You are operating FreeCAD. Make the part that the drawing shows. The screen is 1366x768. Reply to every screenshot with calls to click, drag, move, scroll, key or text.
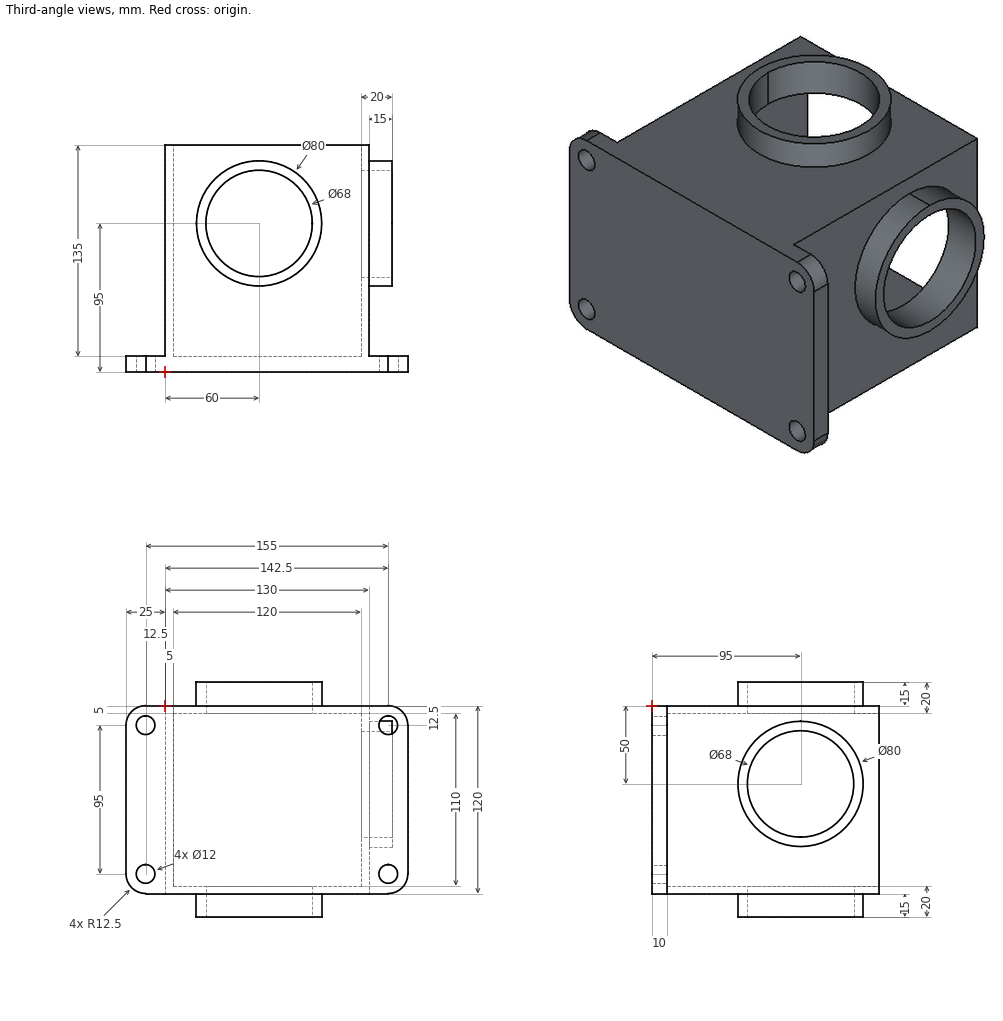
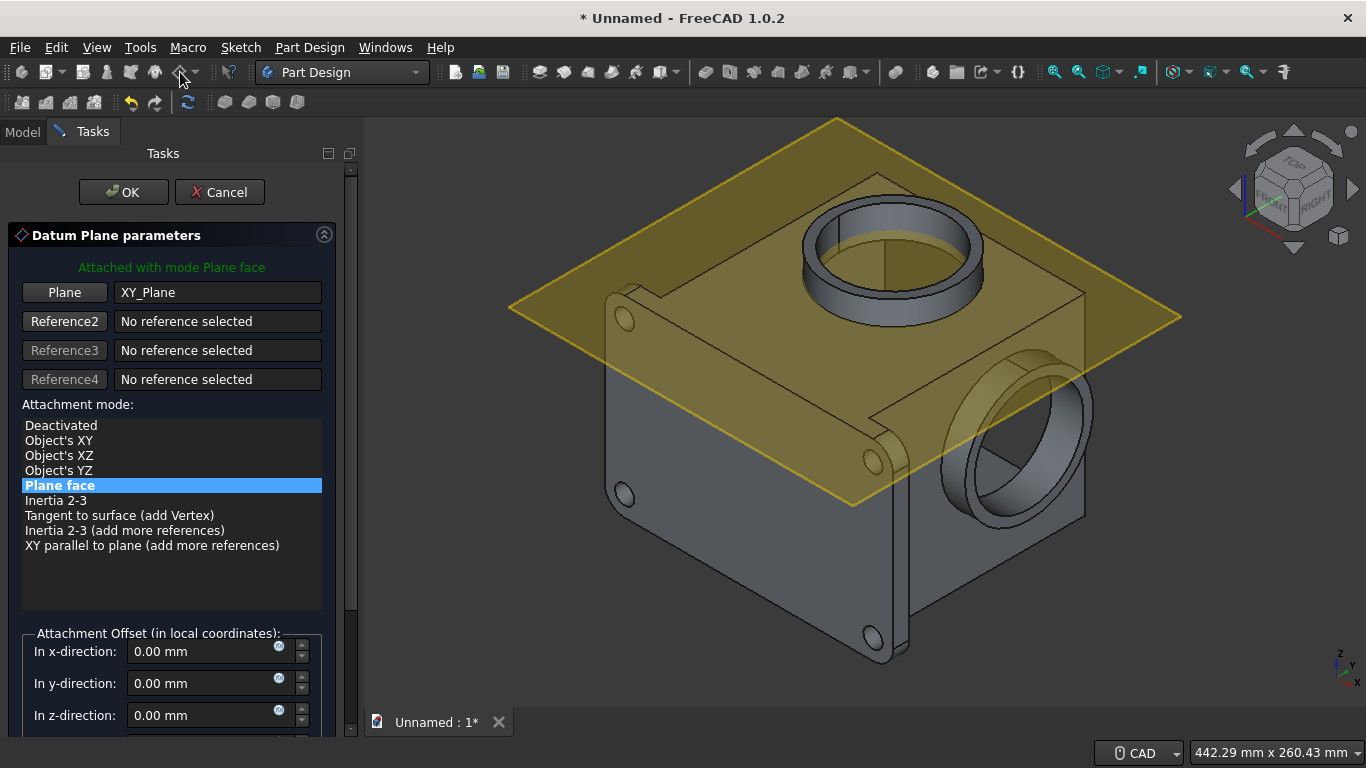
triple_click(210, 715)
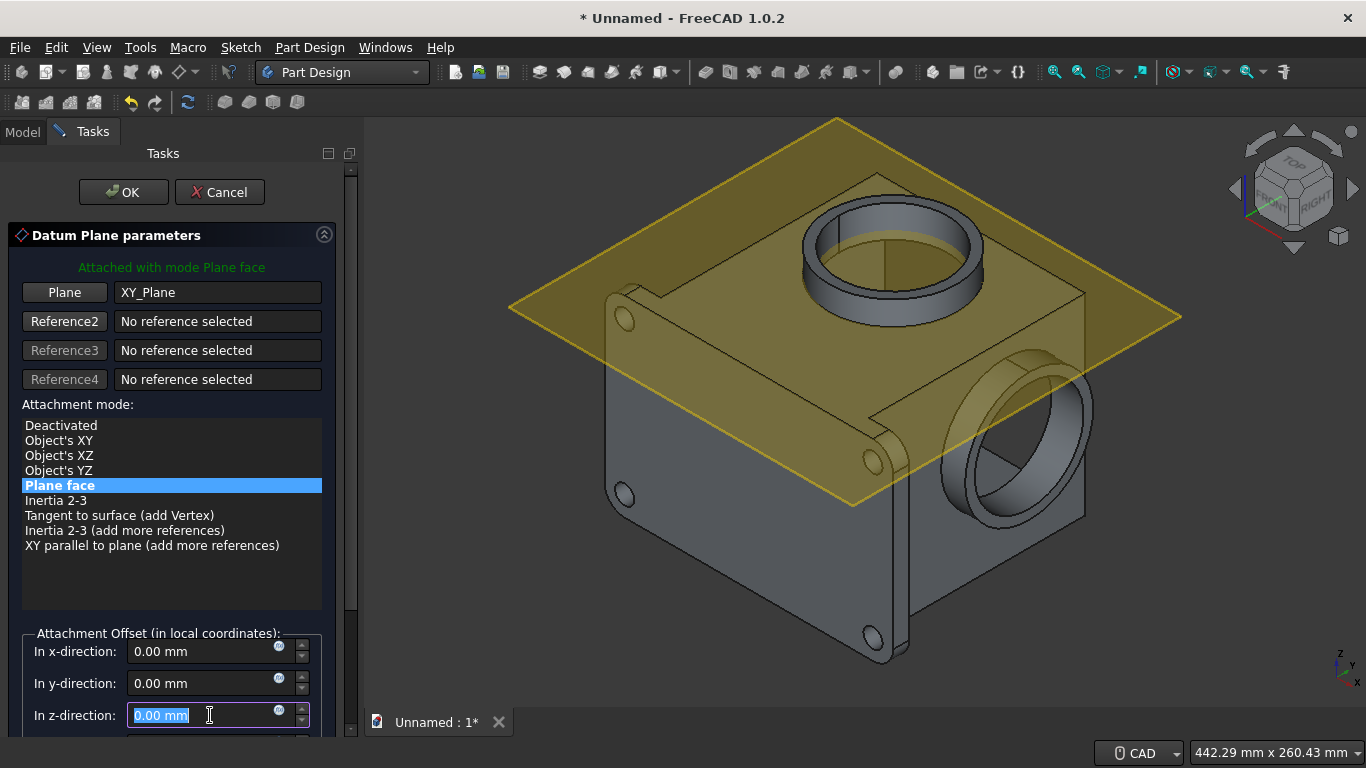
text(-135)
key(Tab)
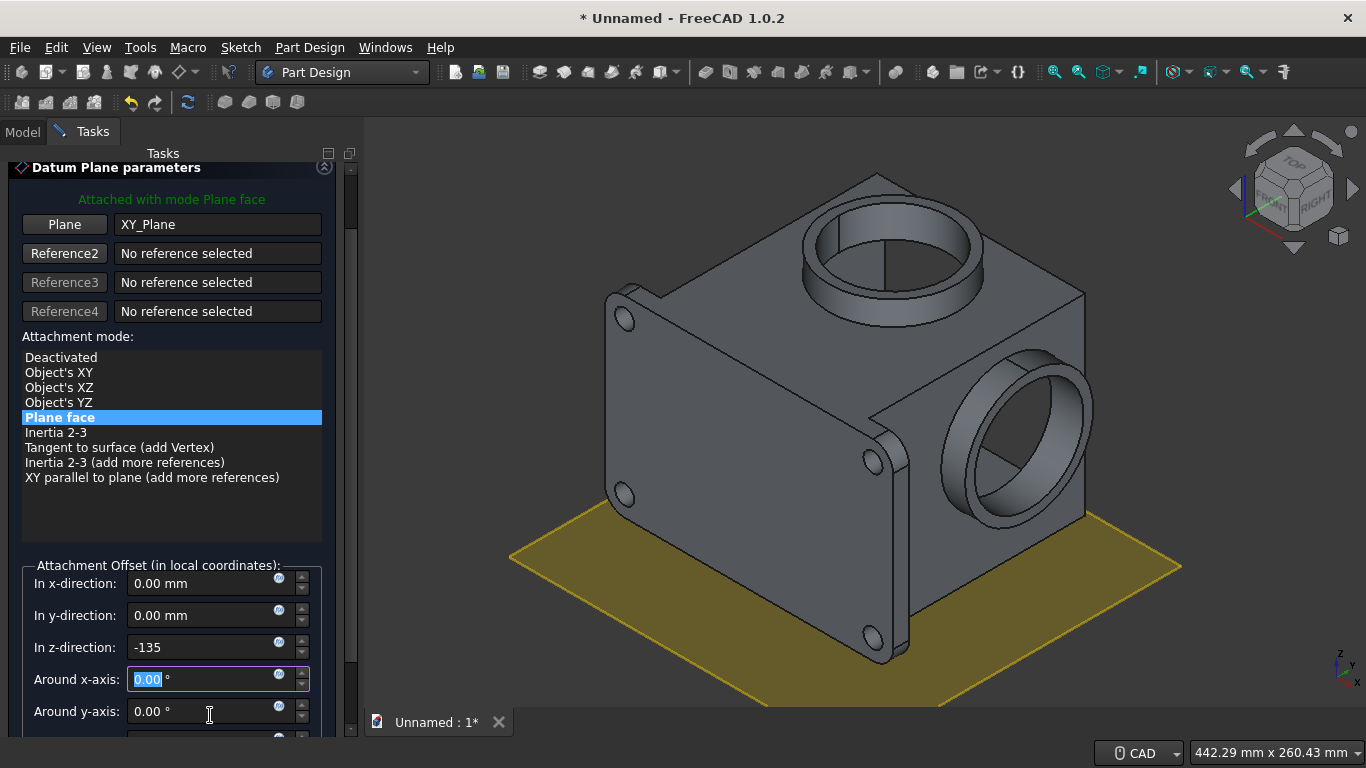
scroll(351, 450, up, 2)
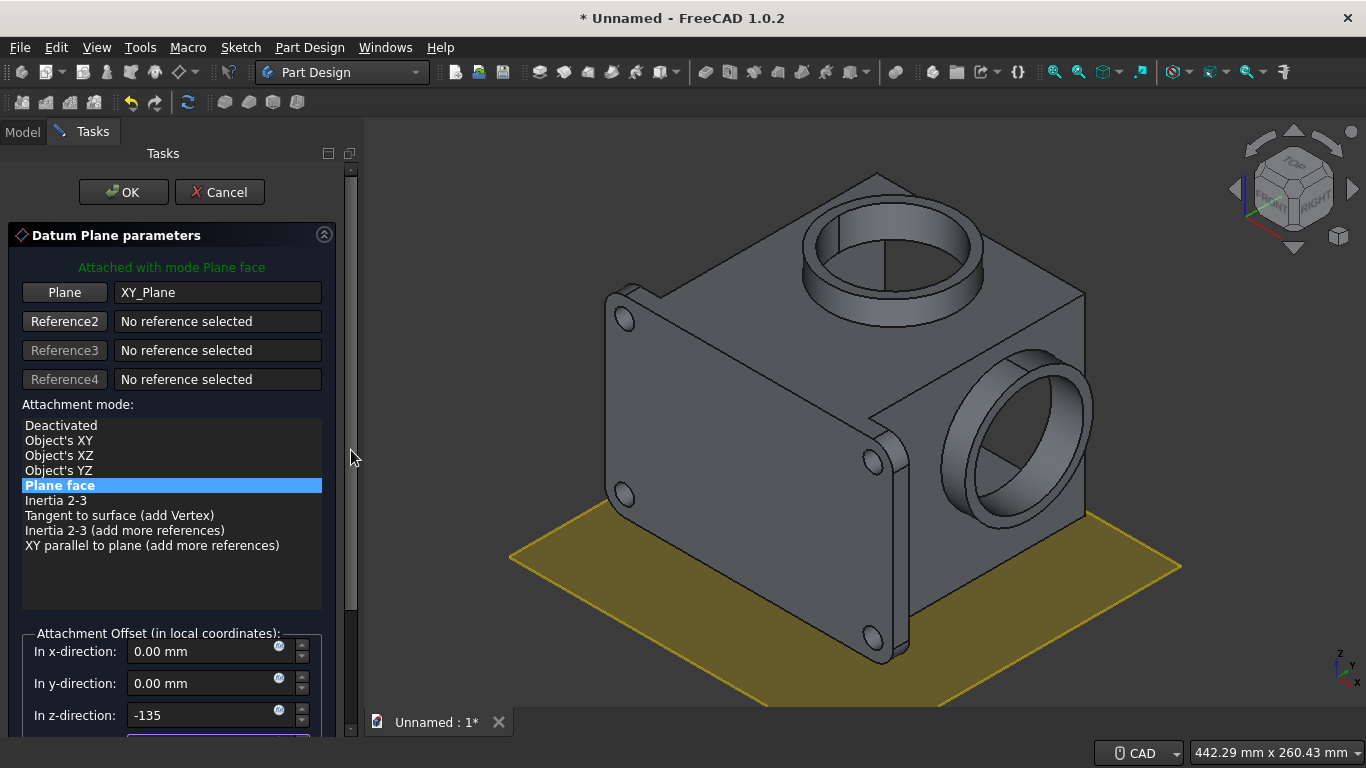
click(124, 192)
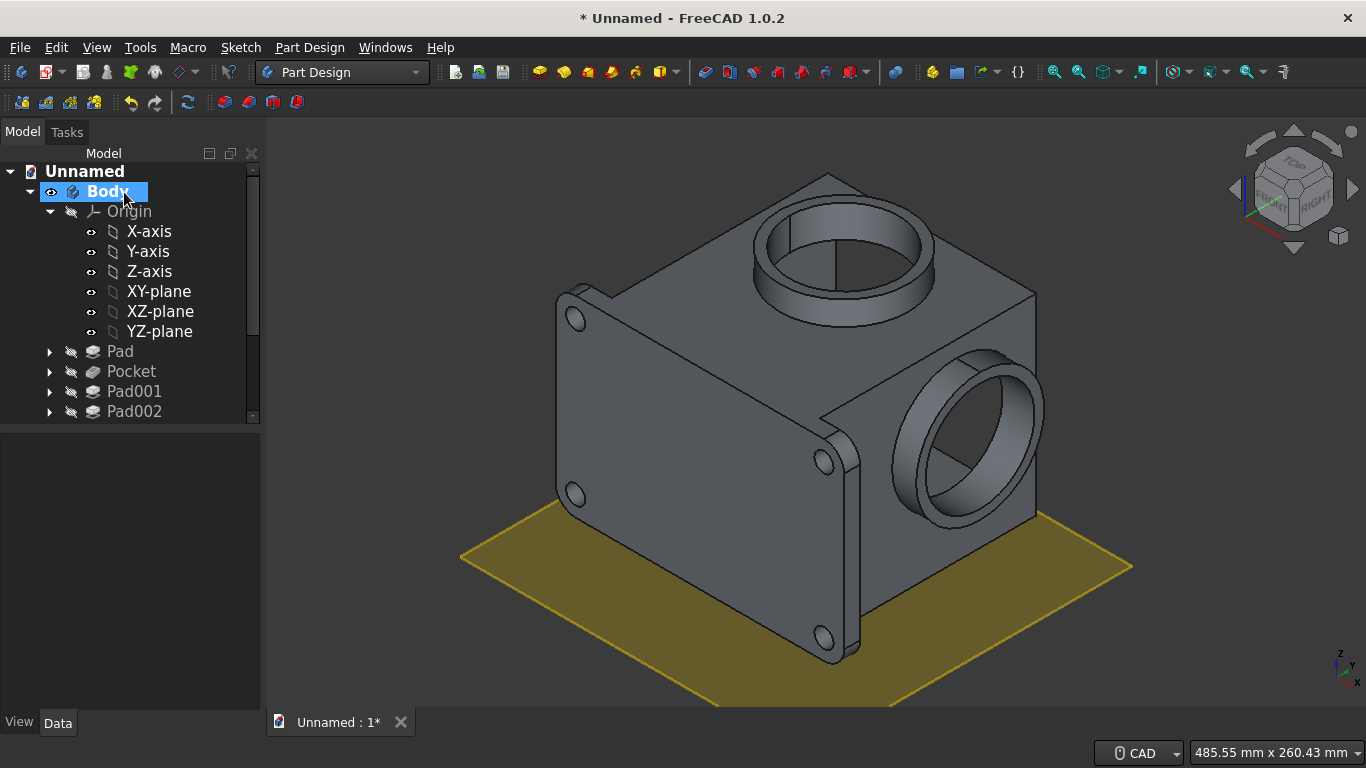
scroll(100, 287, down, 3)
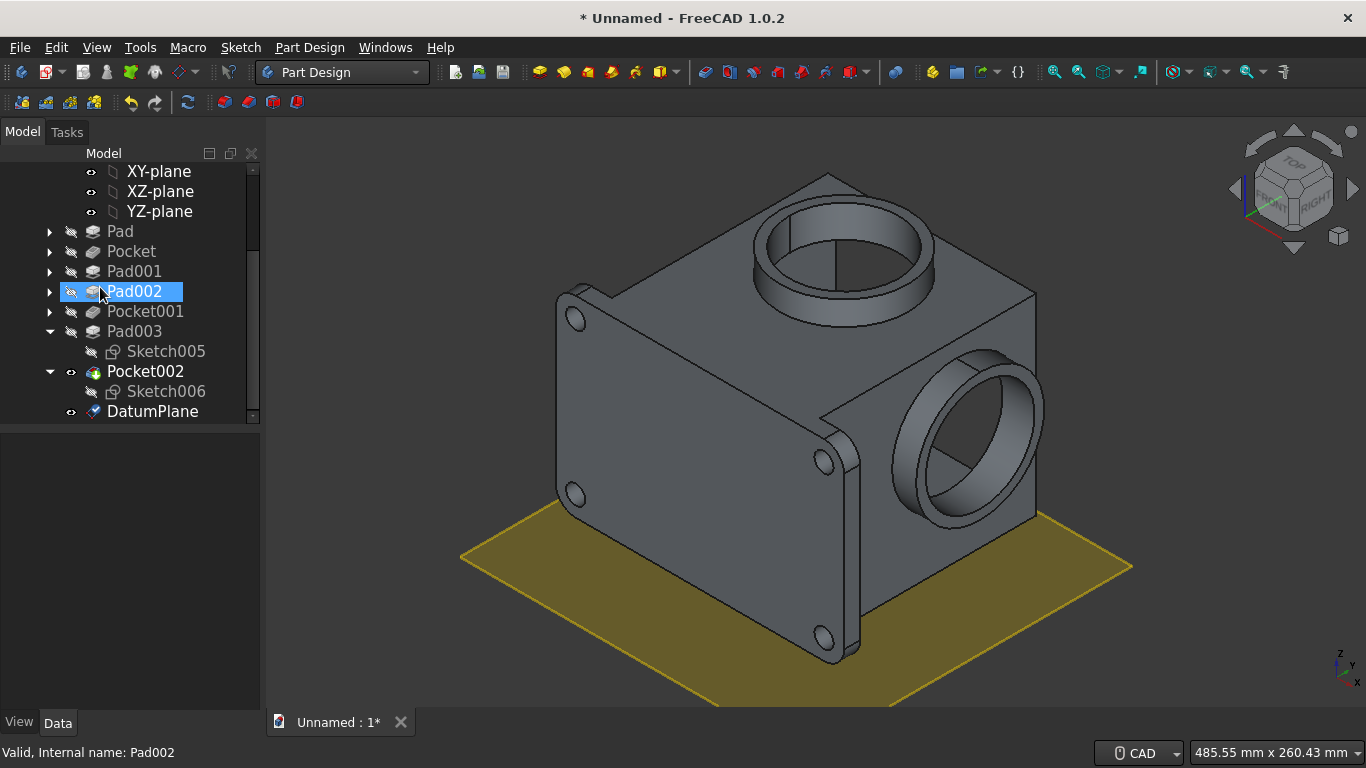
click(116, 412)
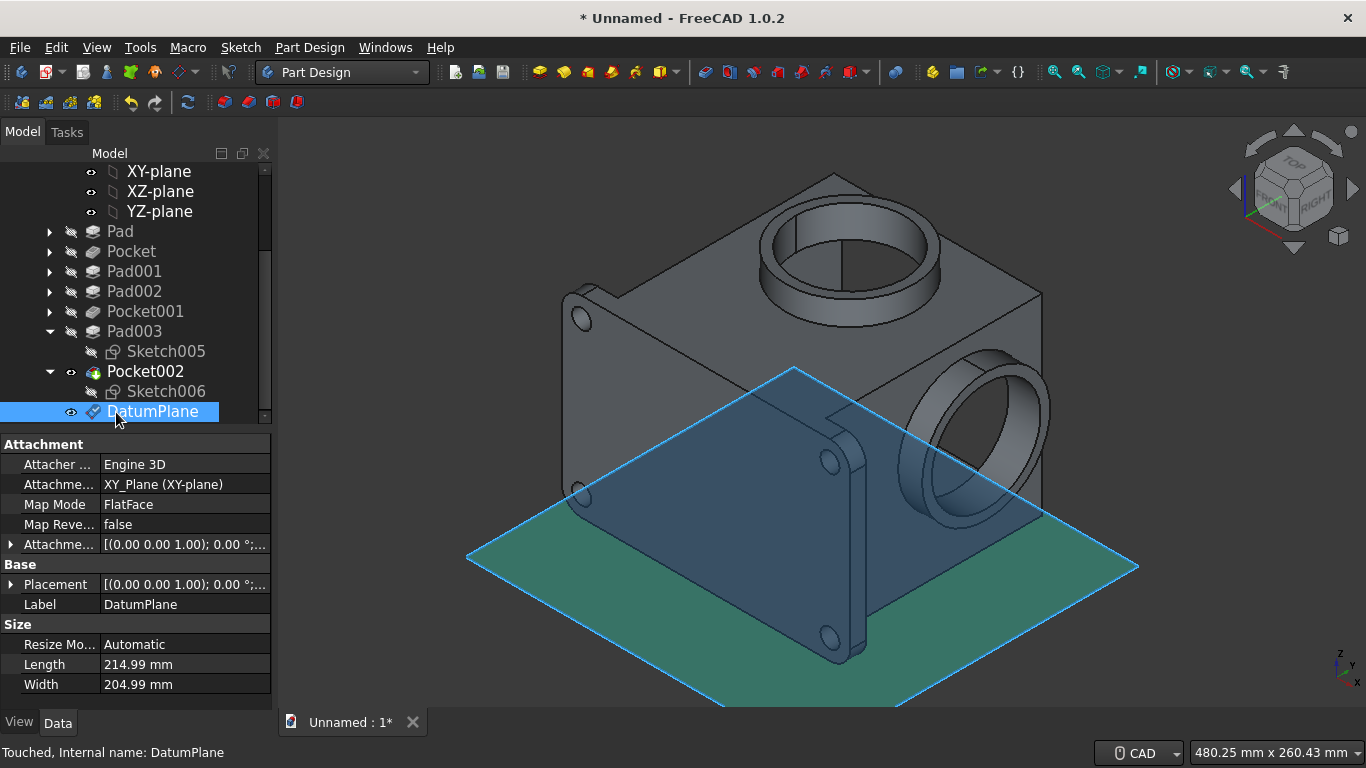
click(46, 72)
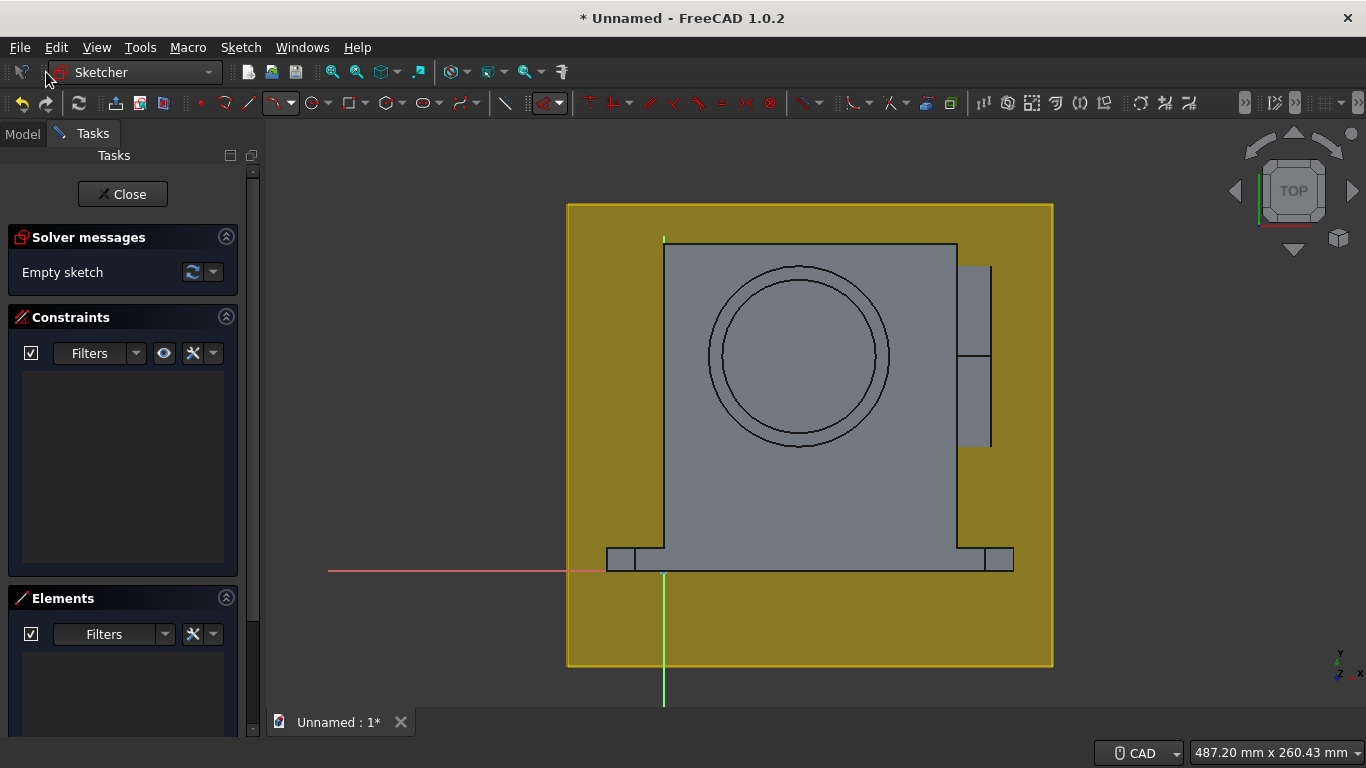
click(164, 104)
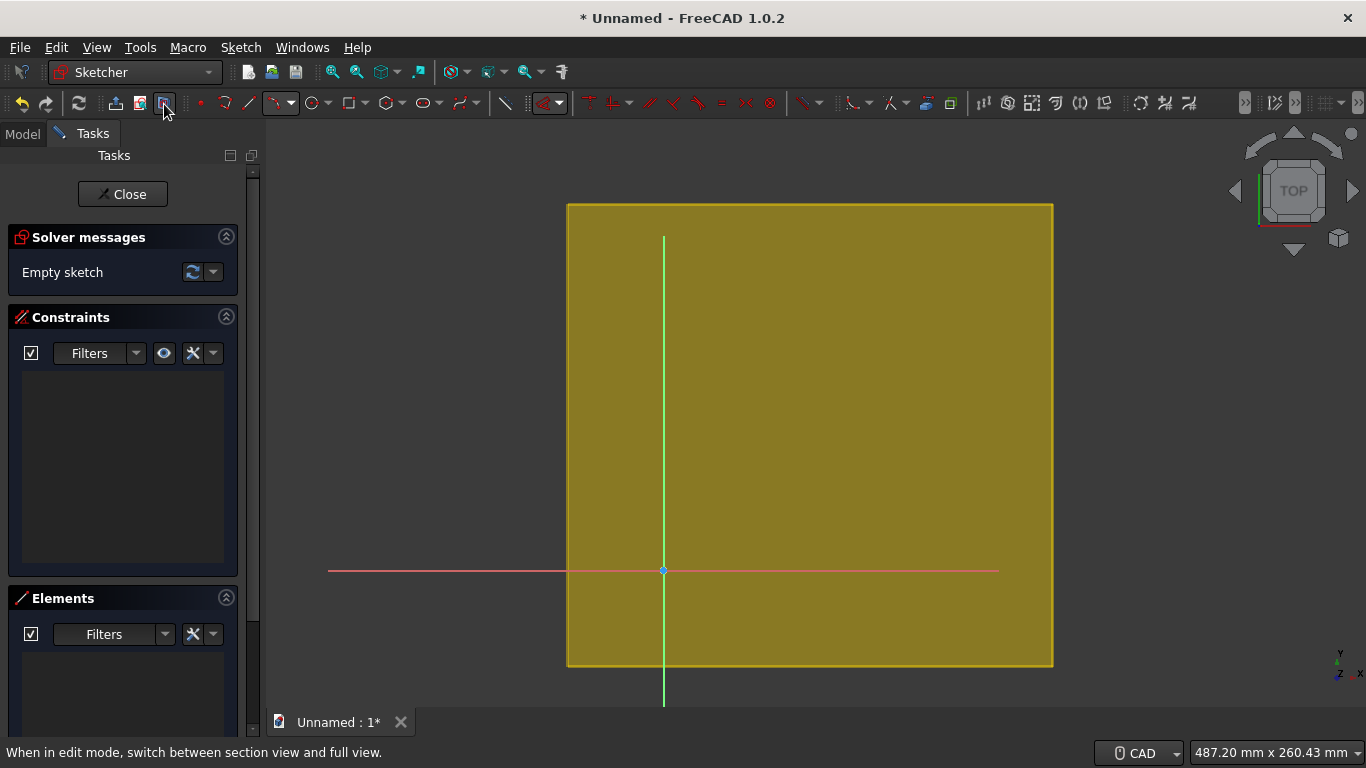
click(312, 104)